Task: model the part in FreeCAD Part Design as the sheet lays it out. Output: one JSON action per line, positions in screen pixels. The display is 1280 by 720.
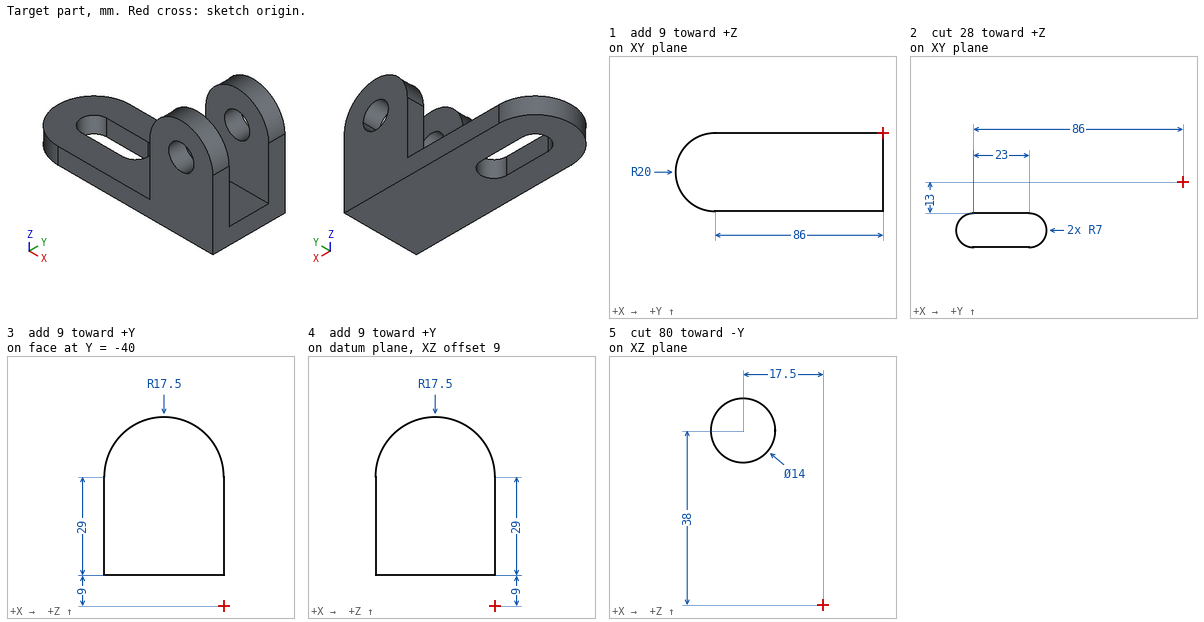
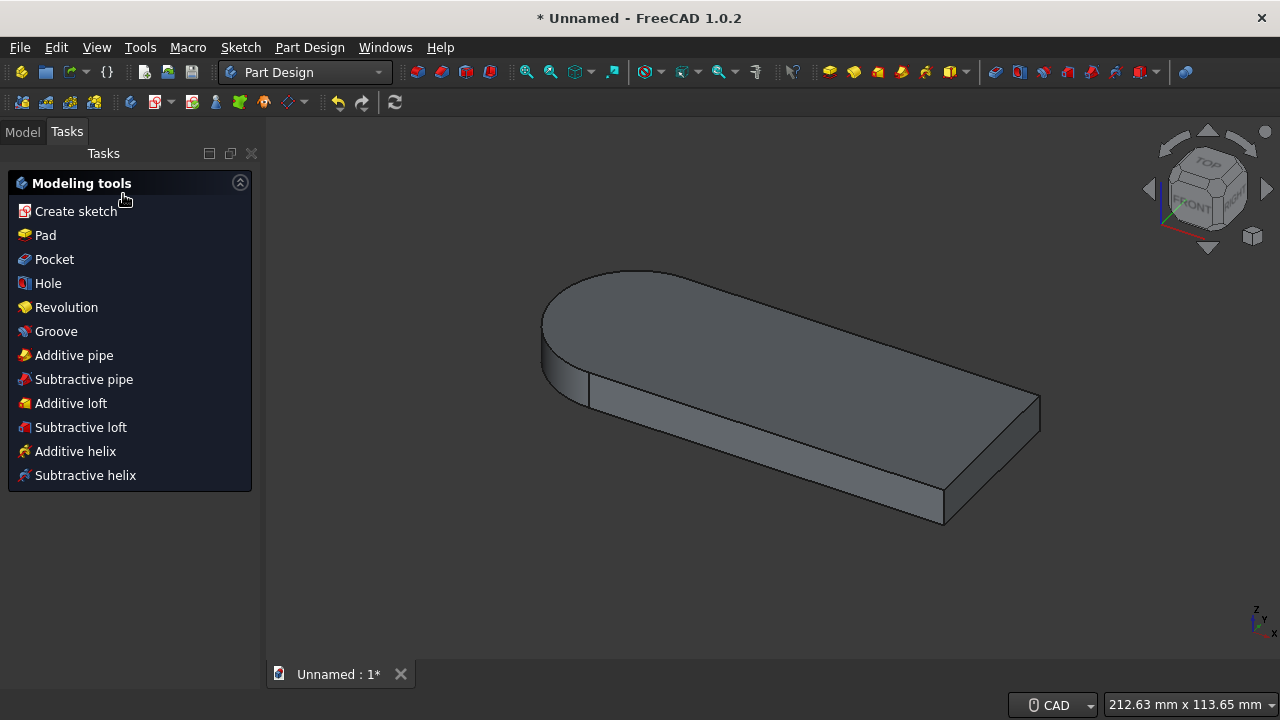
{"action": "left_click", "coordinate": [996, 72]}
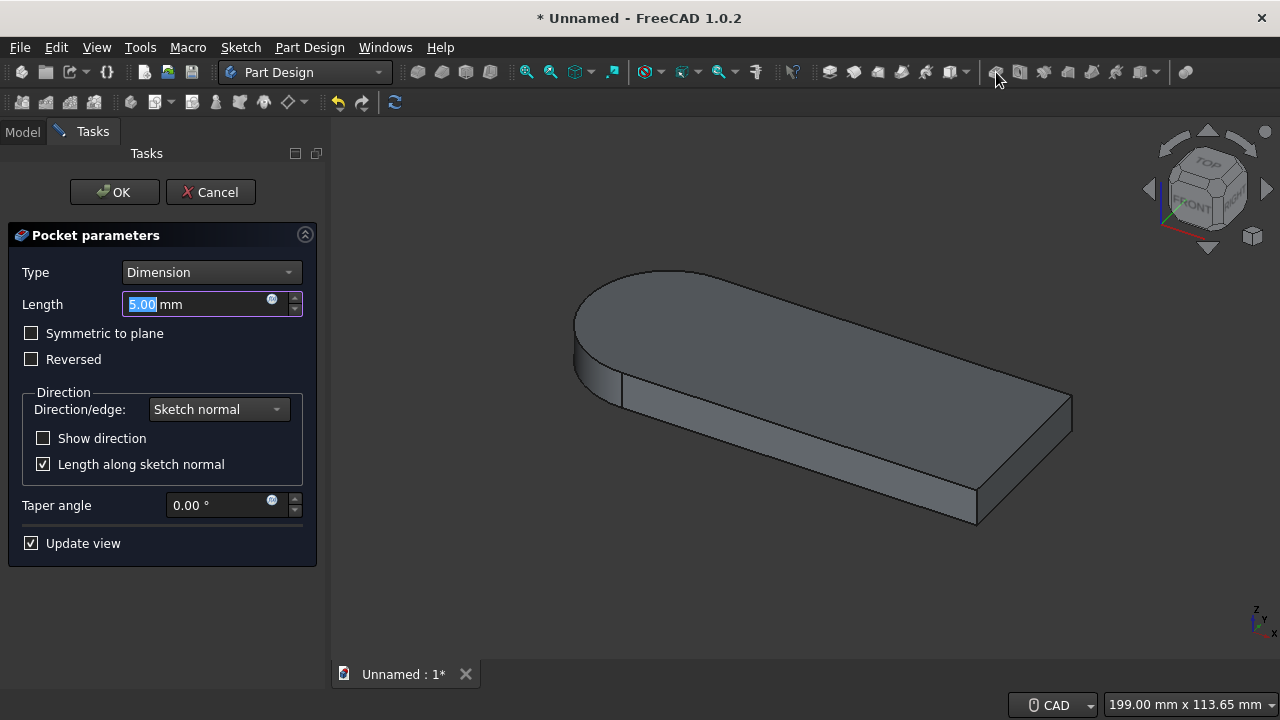
{"action": "type", "text": "28"}
{"action": "key", "text": "Tab"}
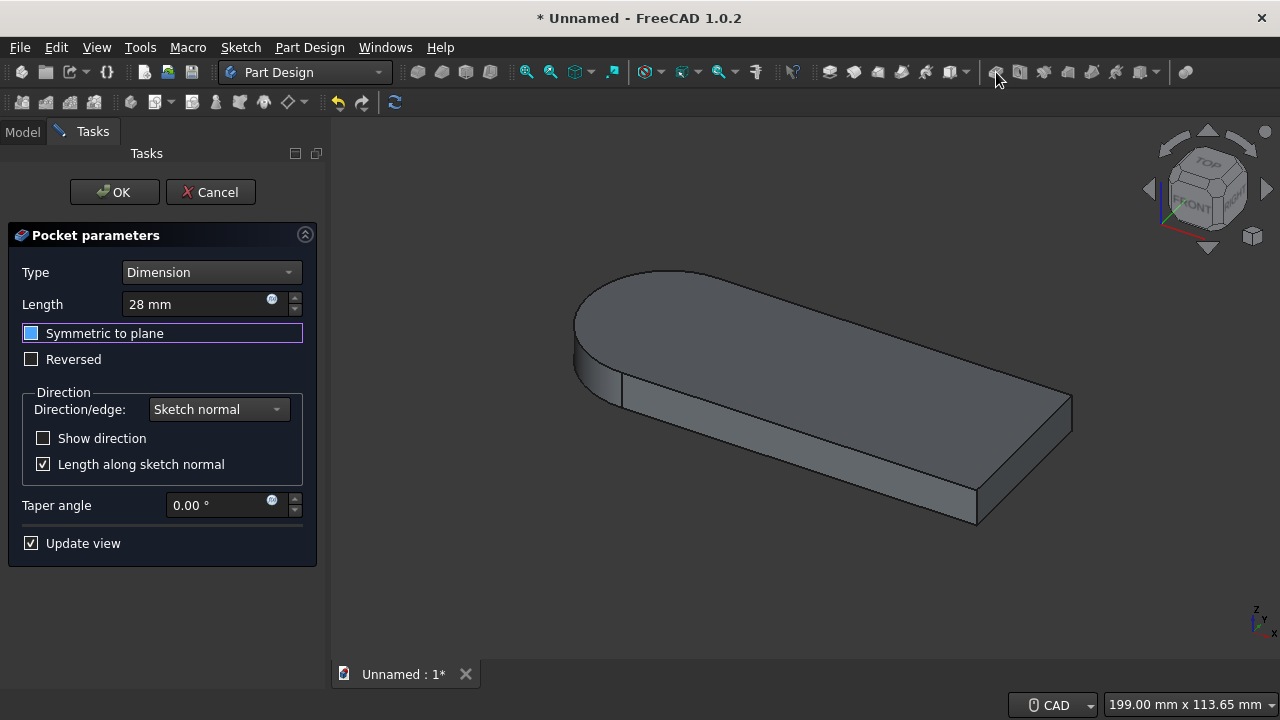
{"action": "left_click", "coordinate": [30, 359]}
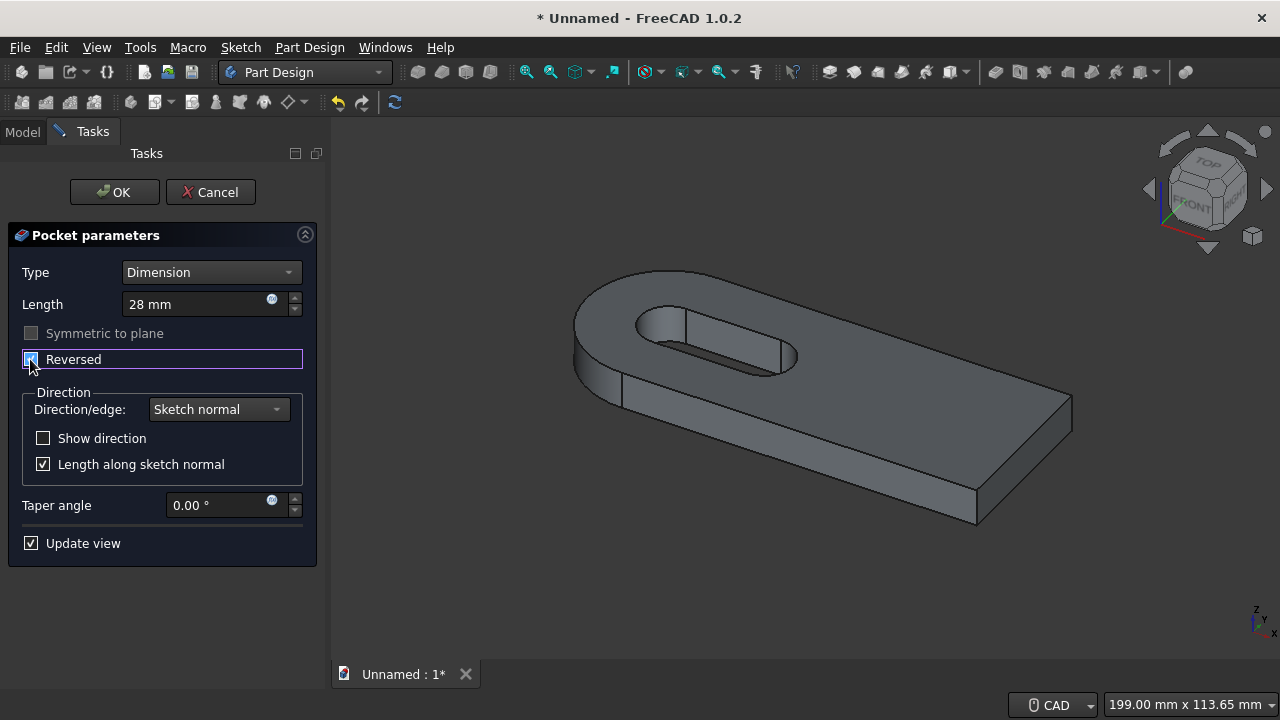
{"action": "left_click", "coordinate": [115, 192]}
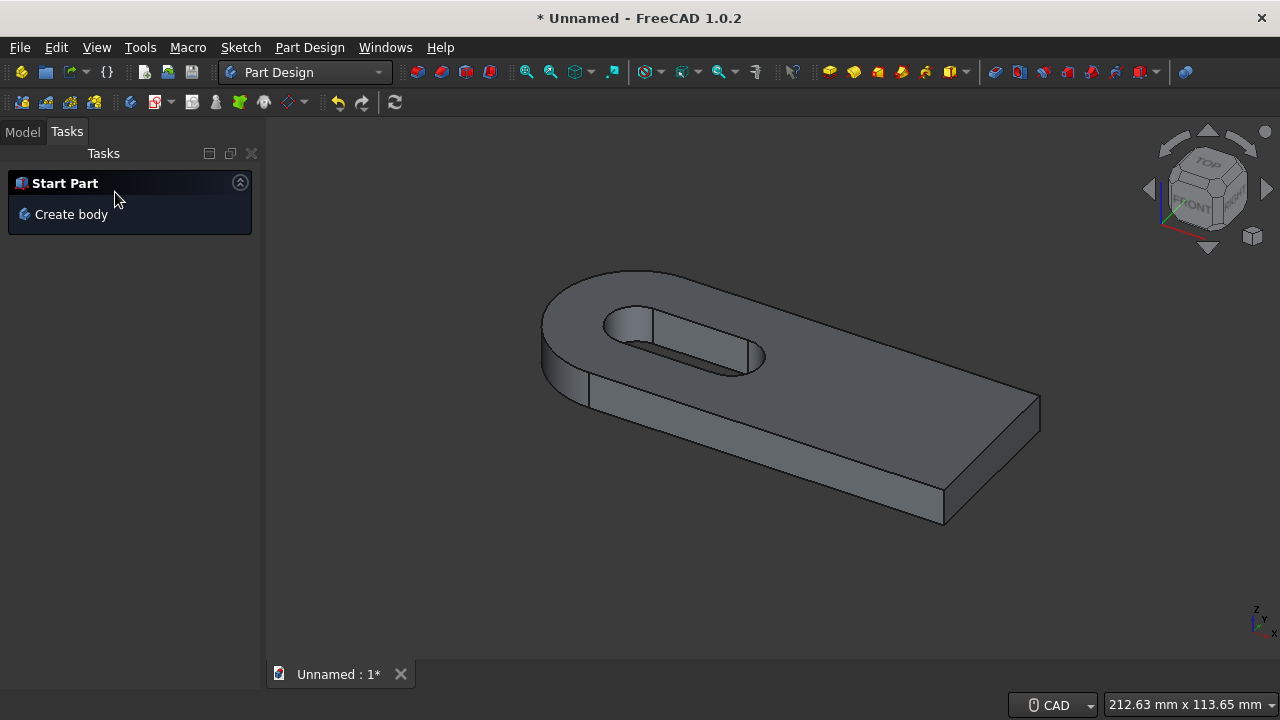
{"action": "left_click", "coordinate": [919, 498]}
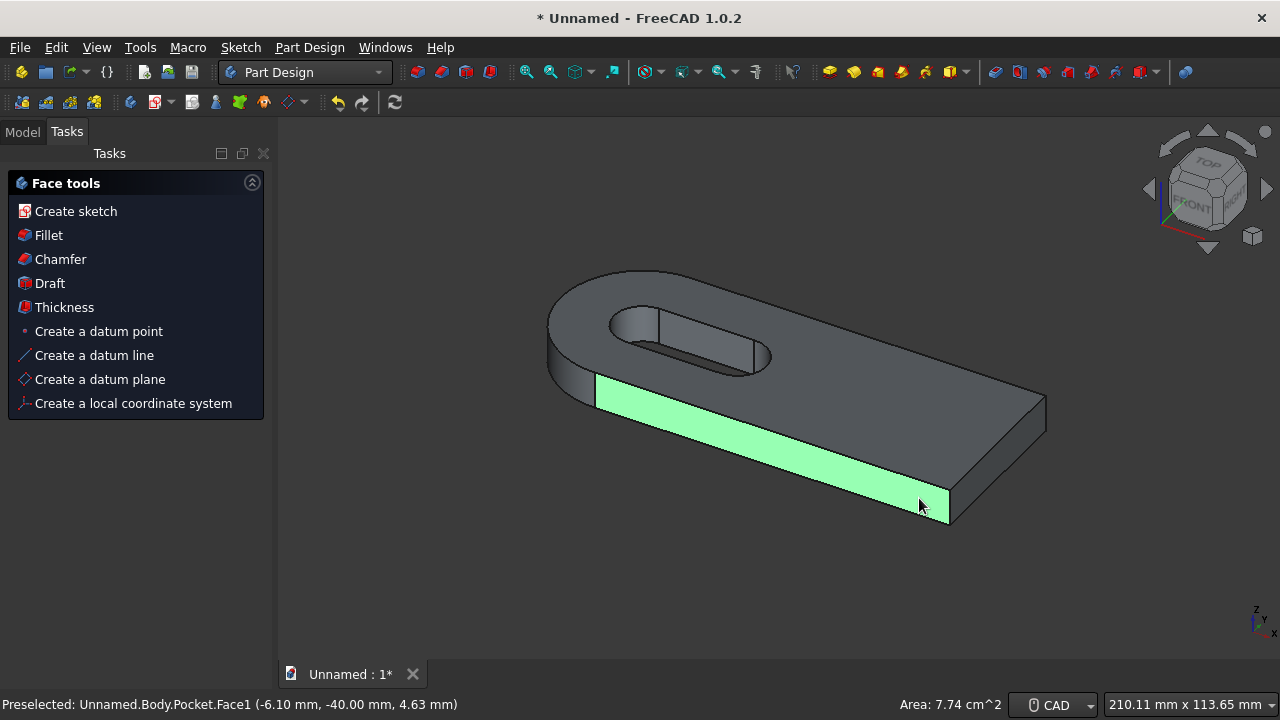
{"action": "left_click", "coordinate": [156, 102]}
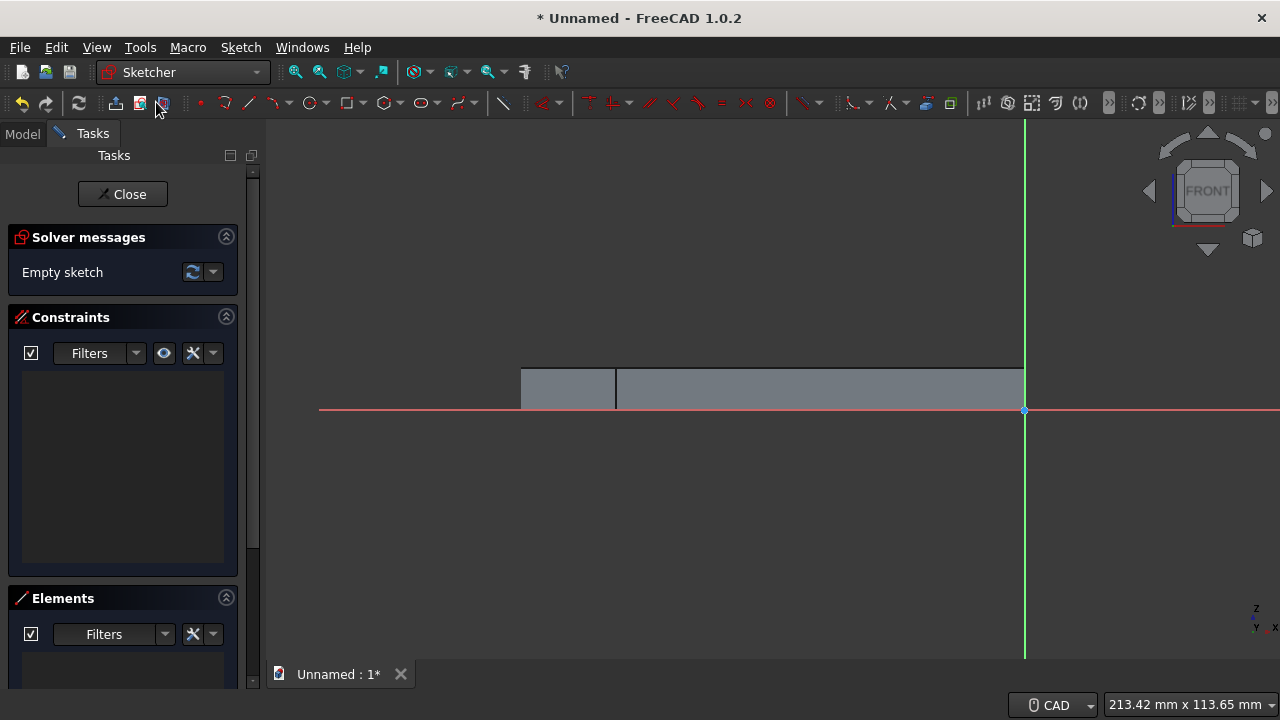
{"action": "scroll", "coordinate": [294, 631], "scroll_direction": "down", "scroll_amount": 1}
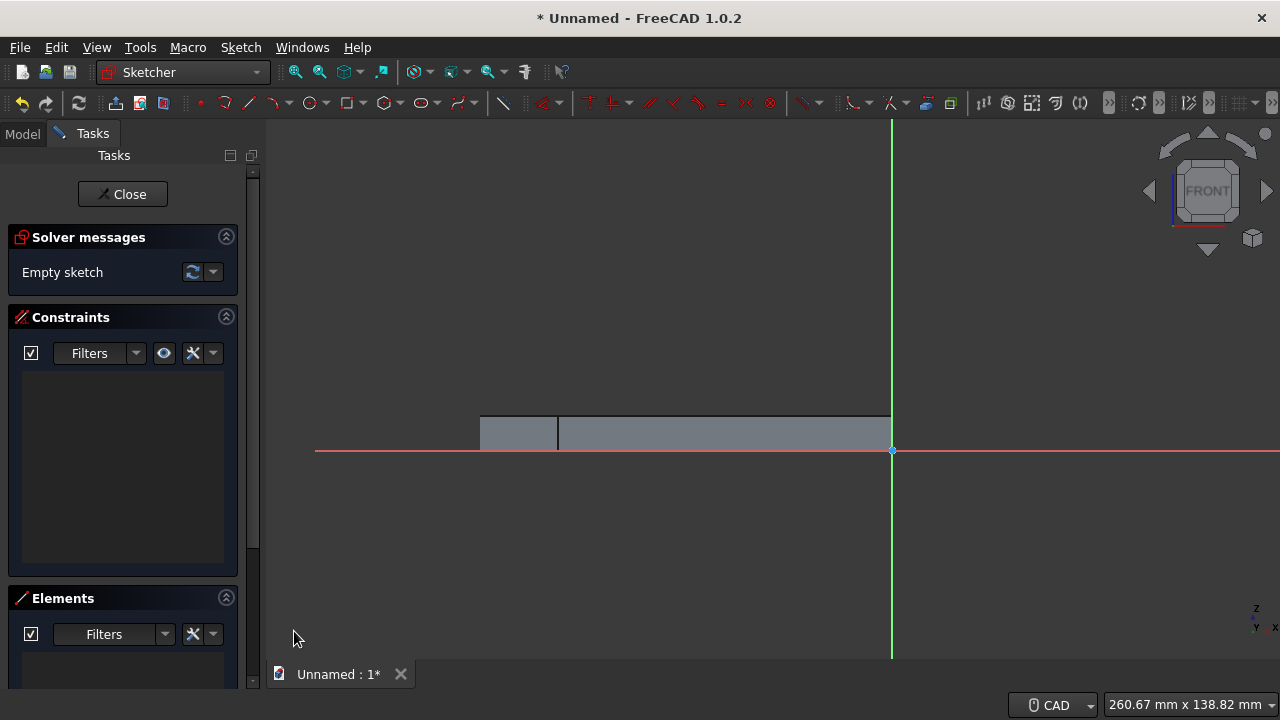
{"action": "scroll", "coordinate": [1068, 248], "scroll_direction": "up", "scroll_amount": 2}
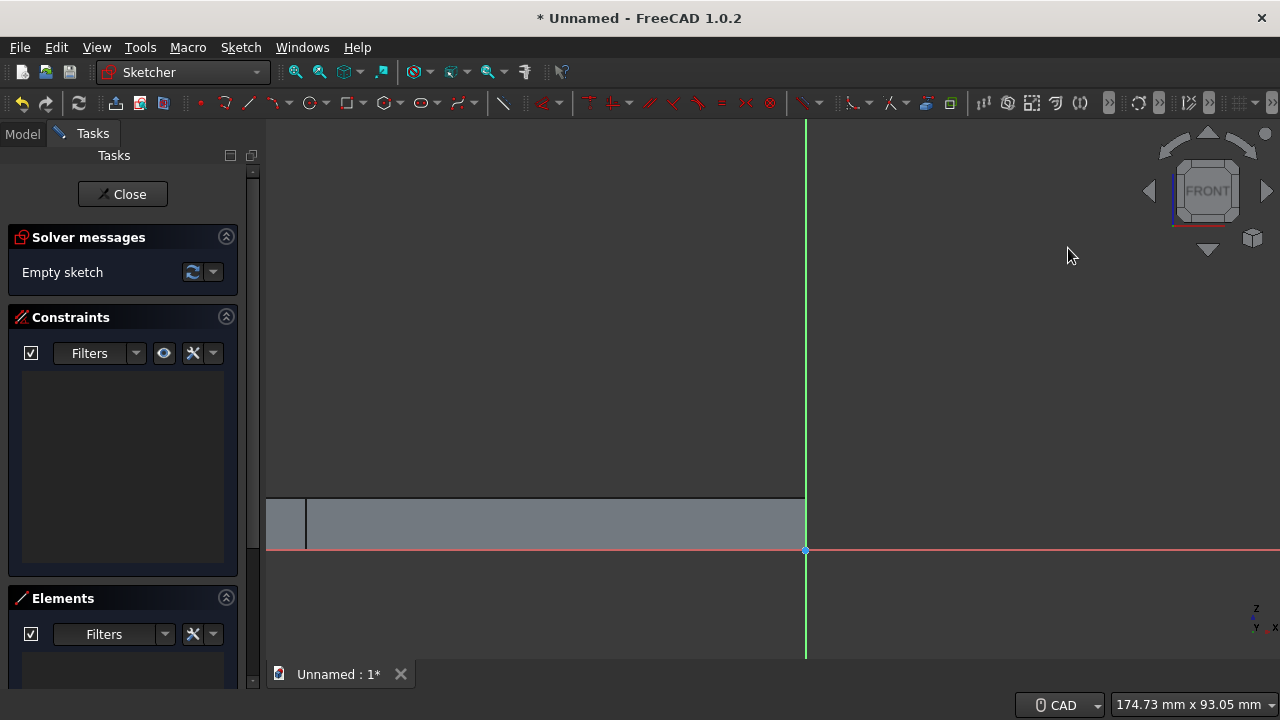
{"action": "left_click", "coordinate": [226, 104]}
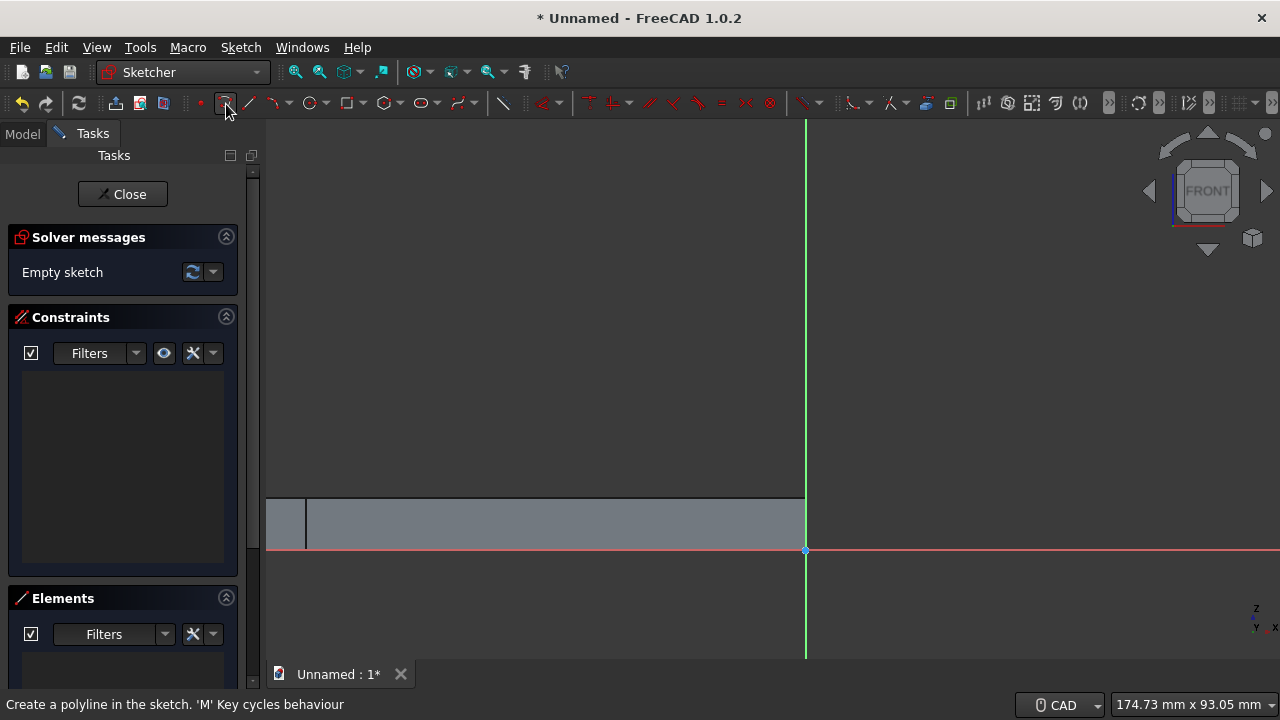
{"action": "left_click", "coordinate": [602, 330]}
{"action": "left_click", "coordinate": [602, 498]}
{"action": "left_click", "coordinate": [806, 498]}
{"action": "left_click", "coordinate": [797, 330]}
{"action": "right_click", "coordinate": [797, 330]}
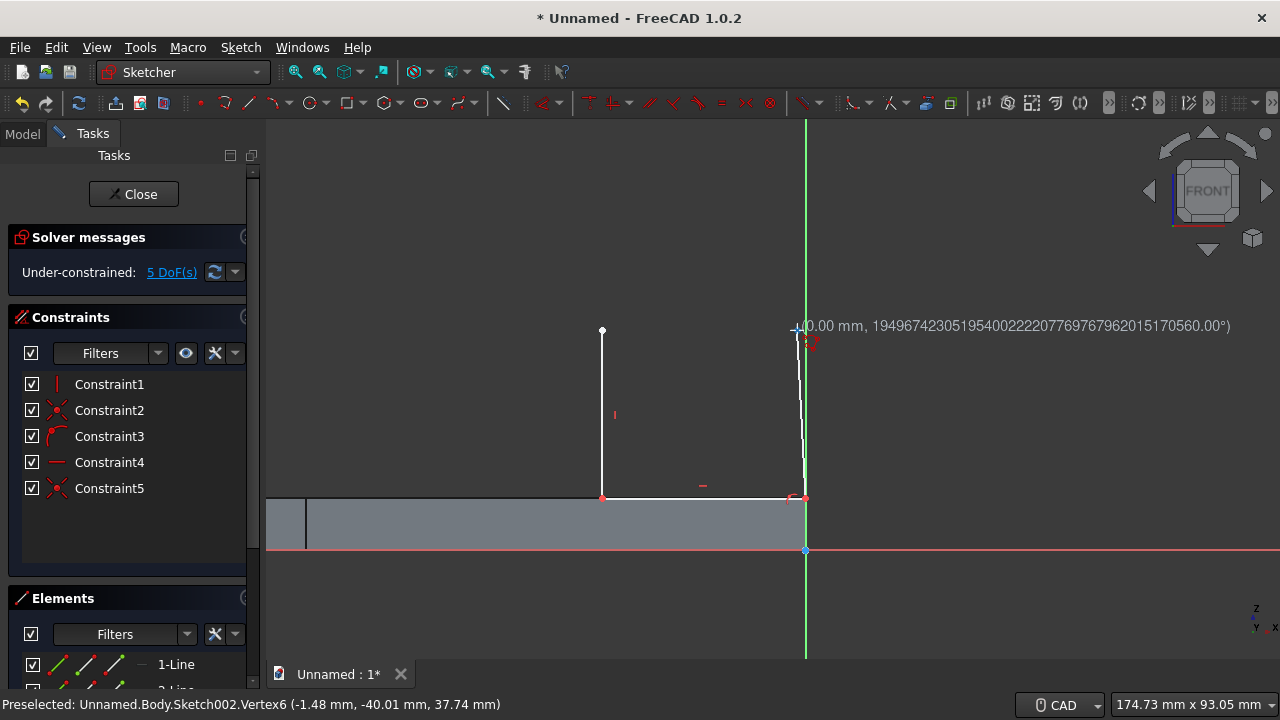
{"action": "left_click", "coordinate": [274, 104]}